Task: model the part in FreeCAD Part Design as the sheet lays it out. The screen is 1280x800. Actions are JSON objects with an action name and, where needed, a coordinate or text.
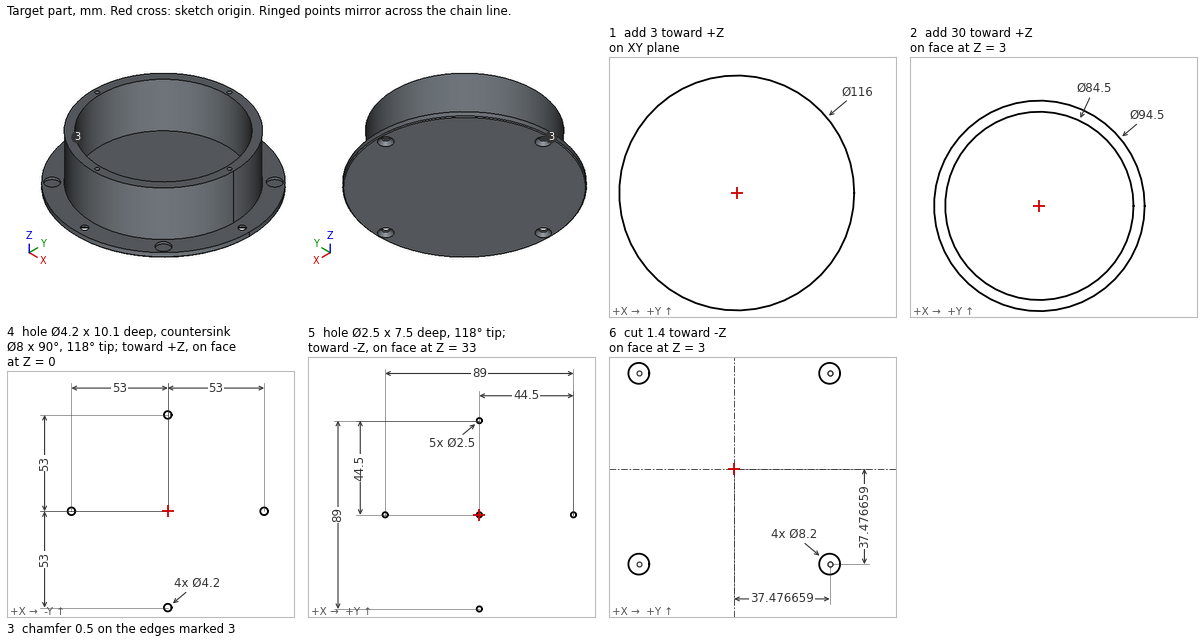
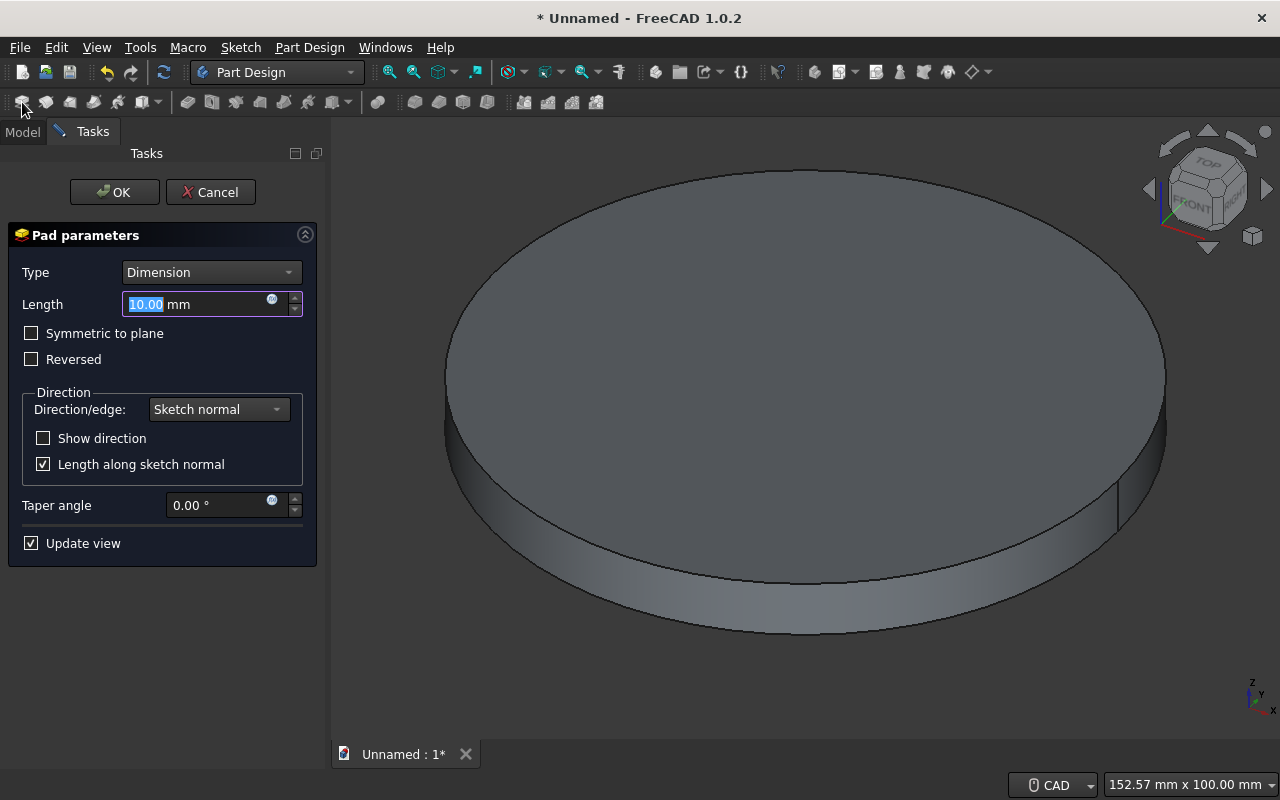
{"action": "type", "text": "3"}
{"action": "key", "text": "Tab"}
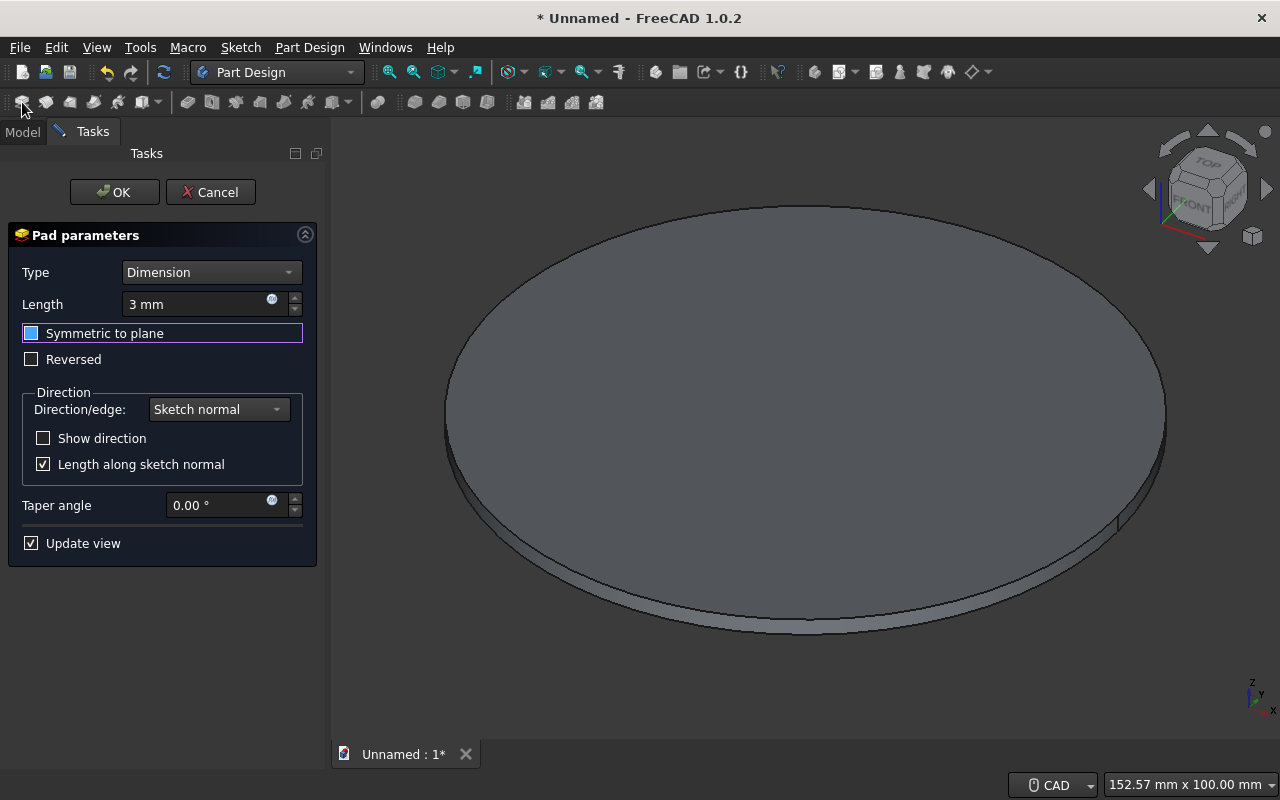
{"action": "left_click", "coordinate": [115, 192]}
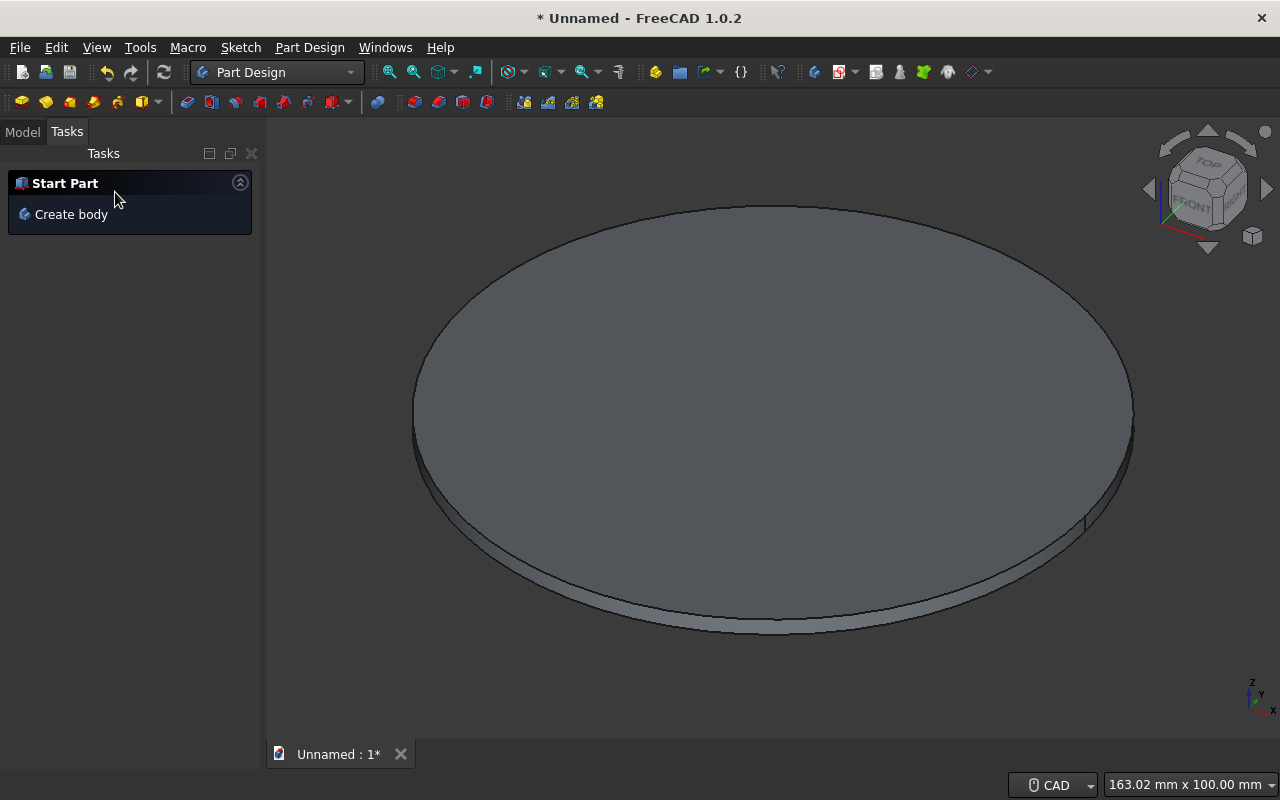
{"action": "left_click", "coordinate": [773, 412]}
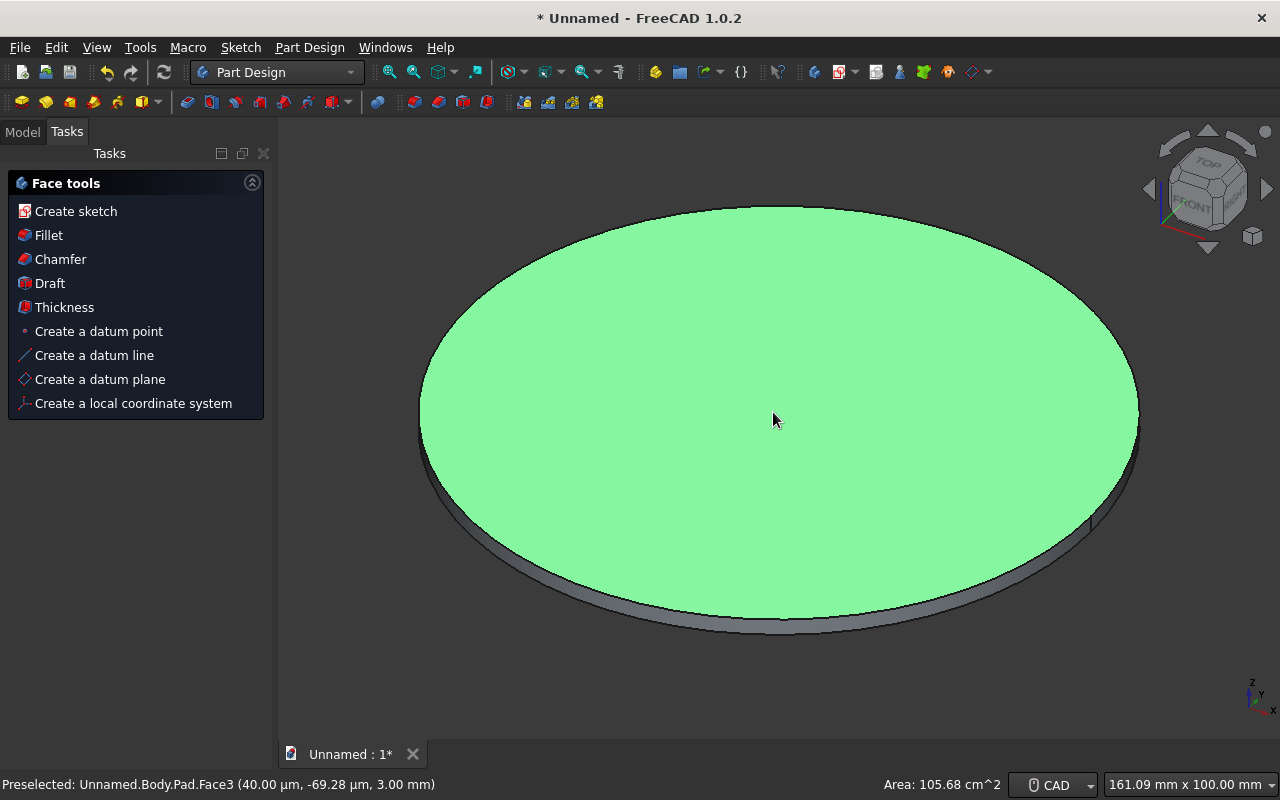
{"action": "left_click", "coordinate": [840, 72]}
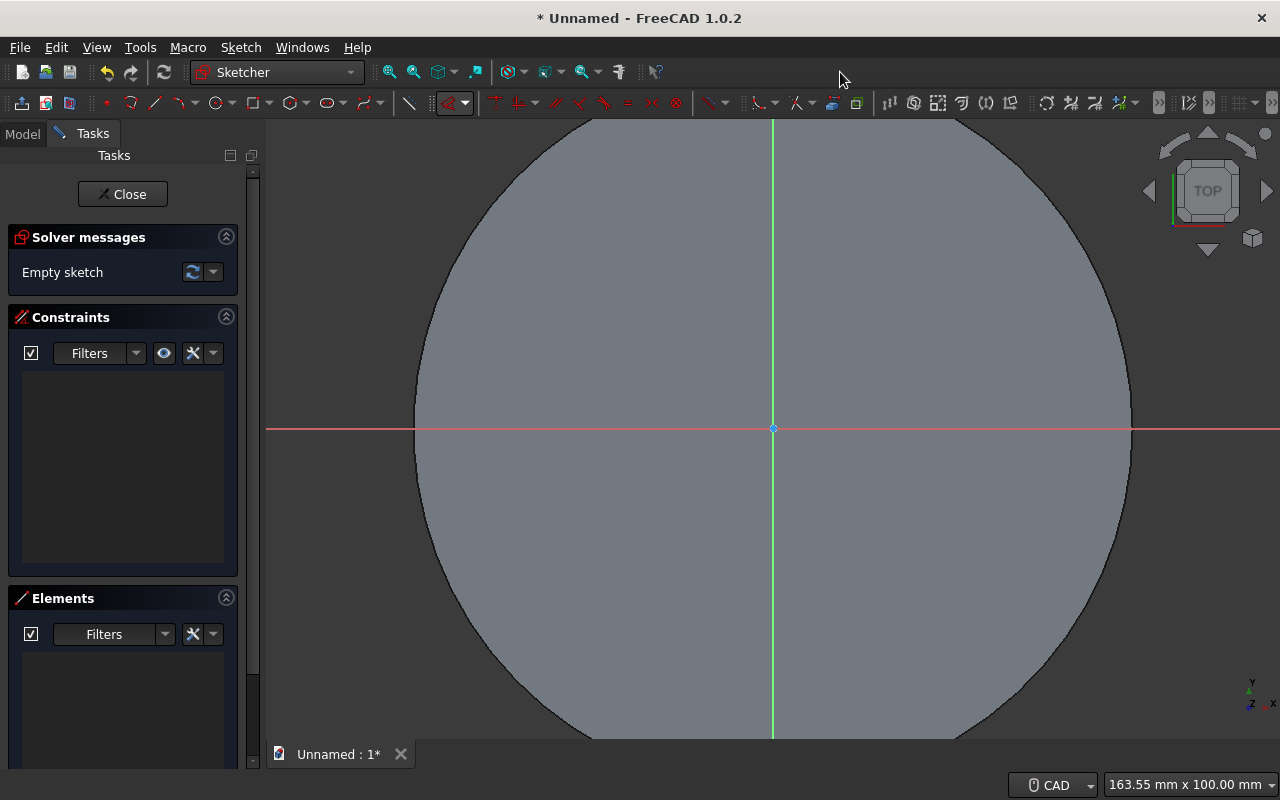
{"action": "scroll", "coordinate": [565, 429], "scroll_direction": "down", "scroll_amount": 2}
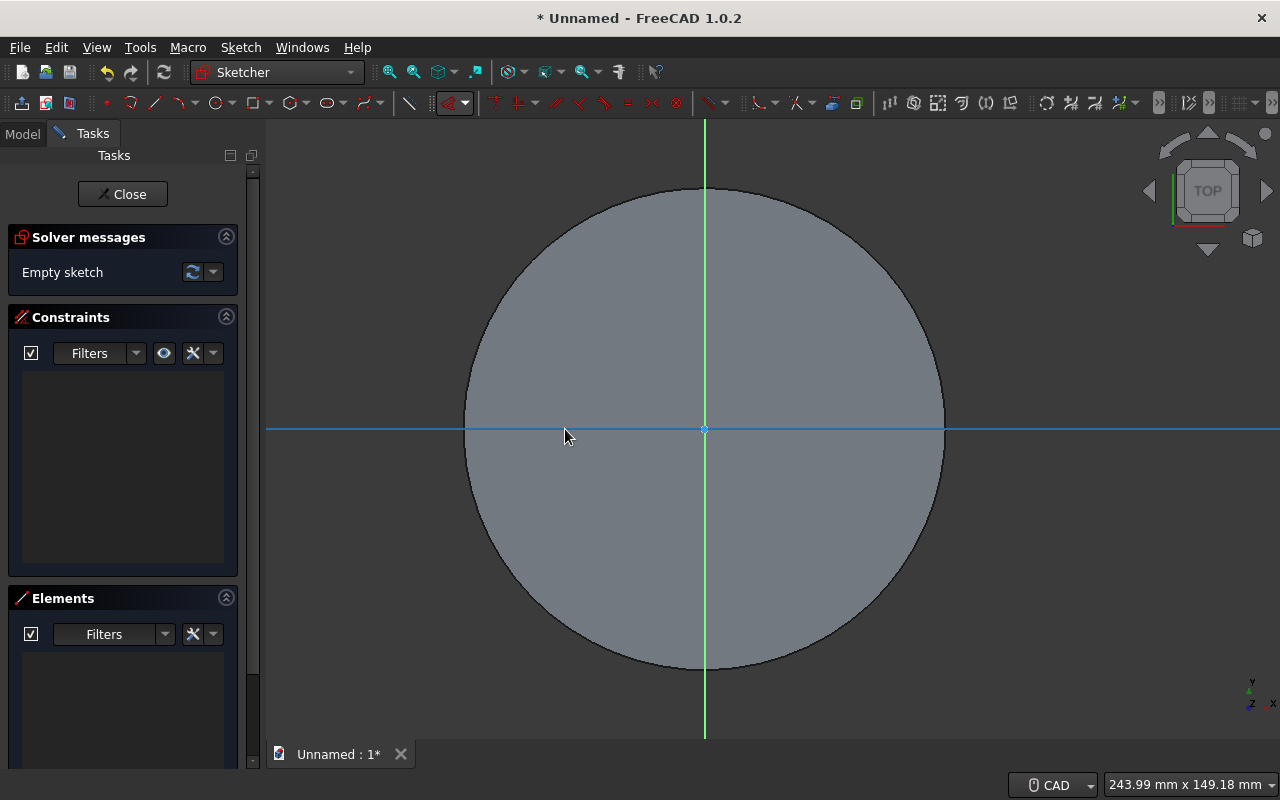
{"action": "left_click", "coordinate": [216, 104]}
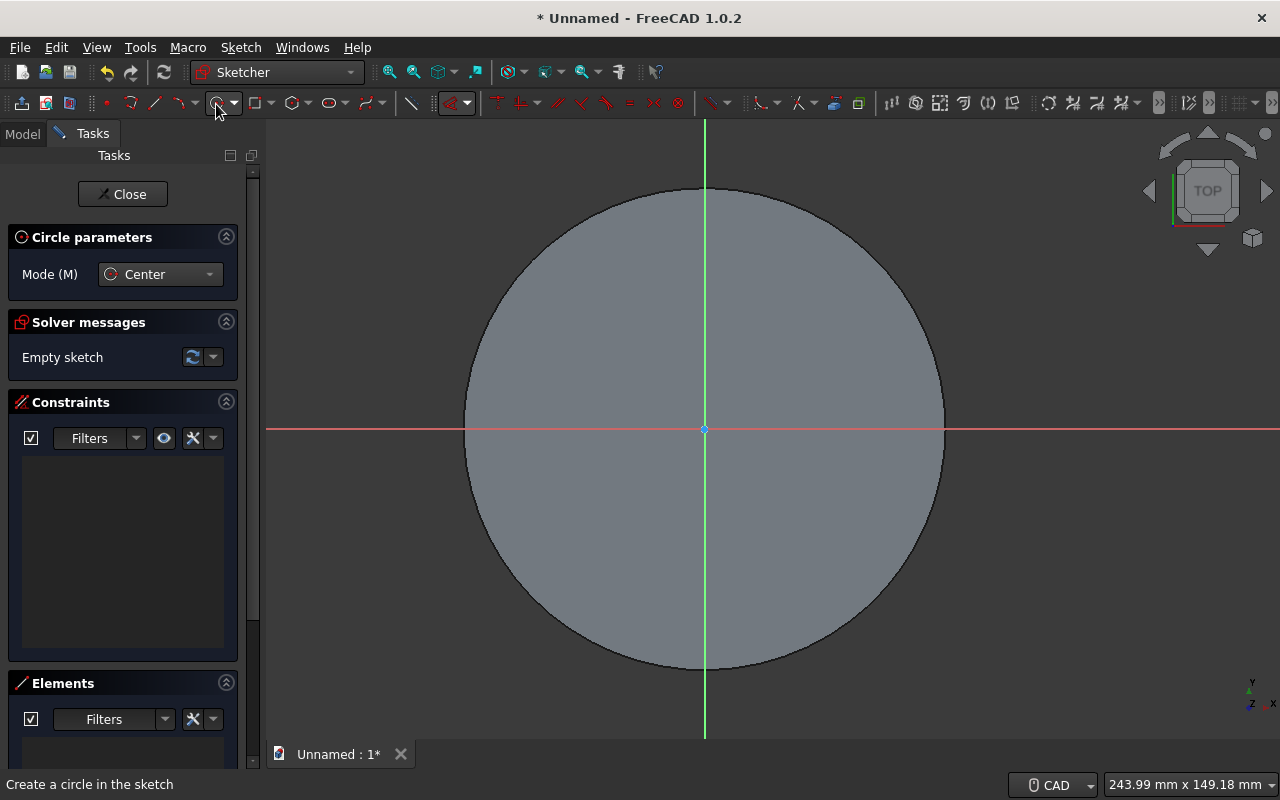
{"action": "left_click", "coordinate": [705, 429]}
{"action": "mouse_move", "coordinate": [843, 290]}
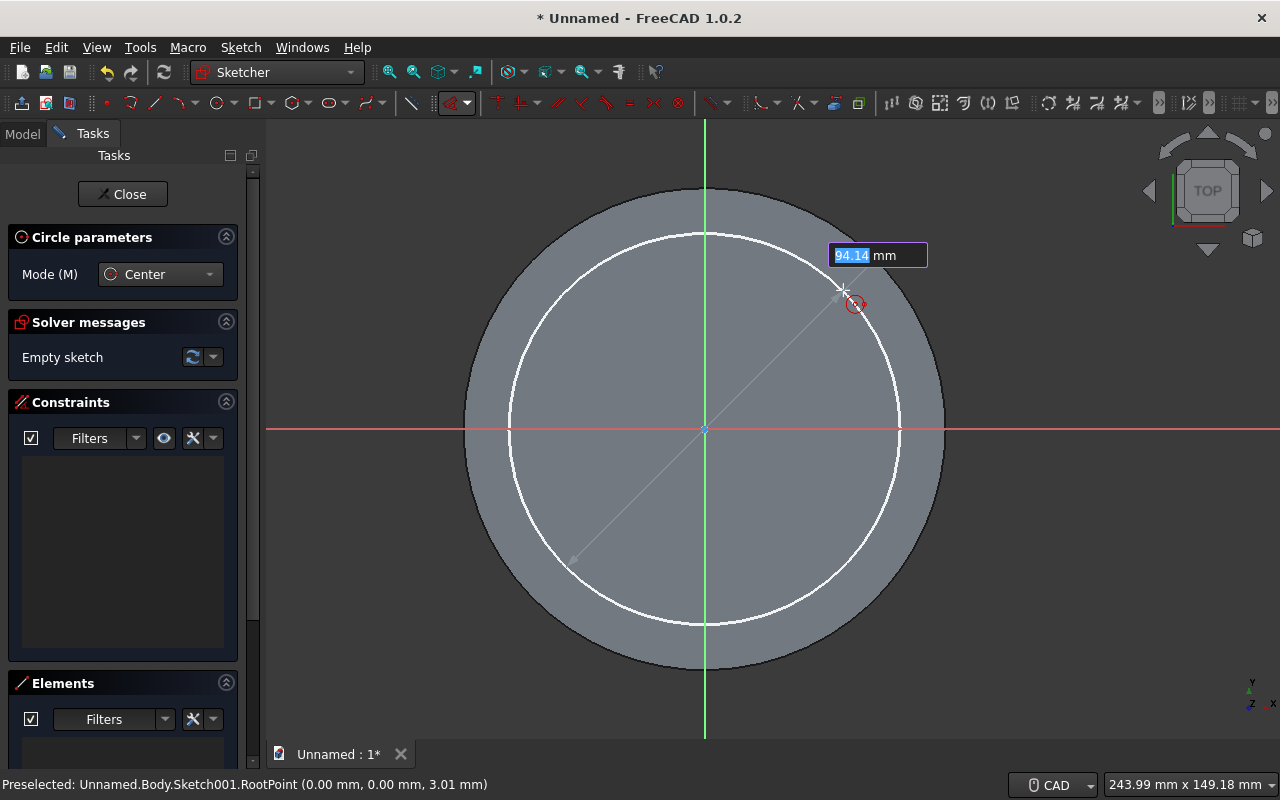
{"action": "type", "text": "94.5"}
{"action": "key", "text": "Return"}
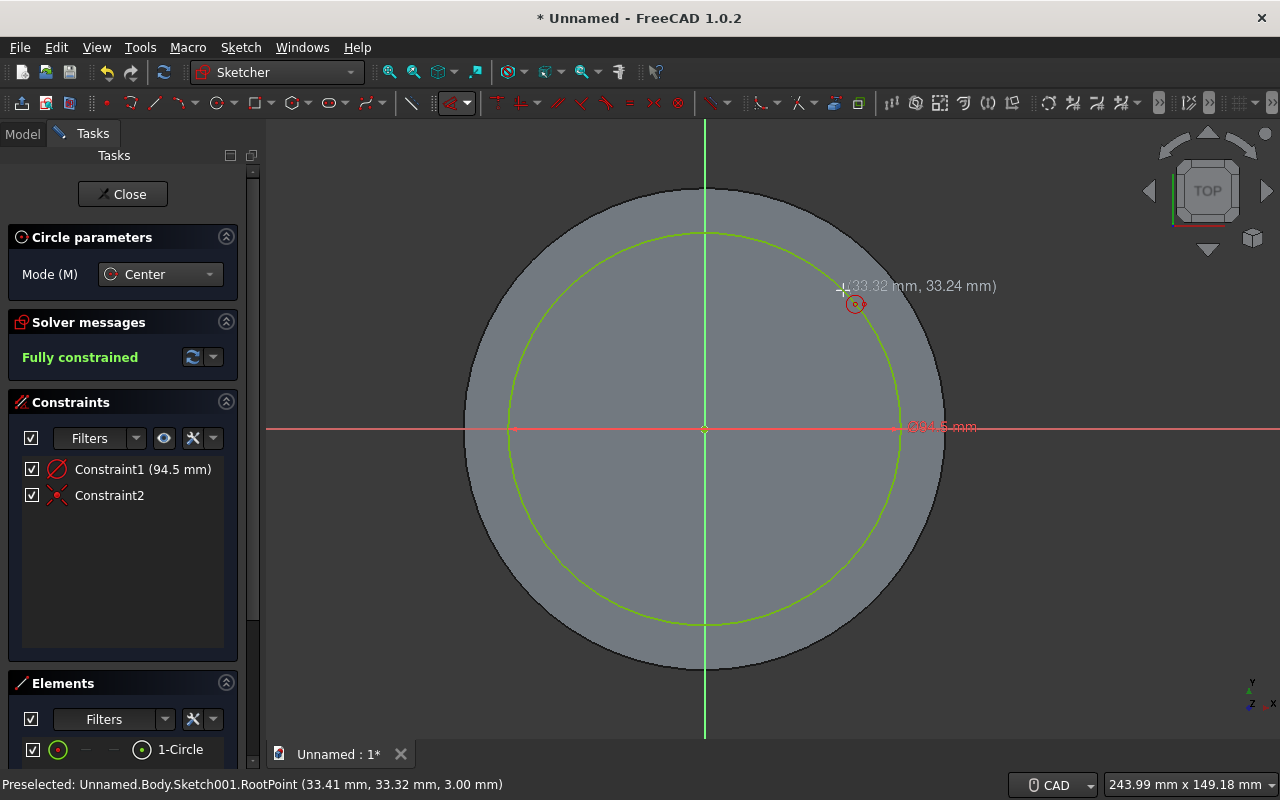
{"action": "left_click", "coordinate": [705, 429]}
{"action": "mouse_move", "coordinate": [829, 305]}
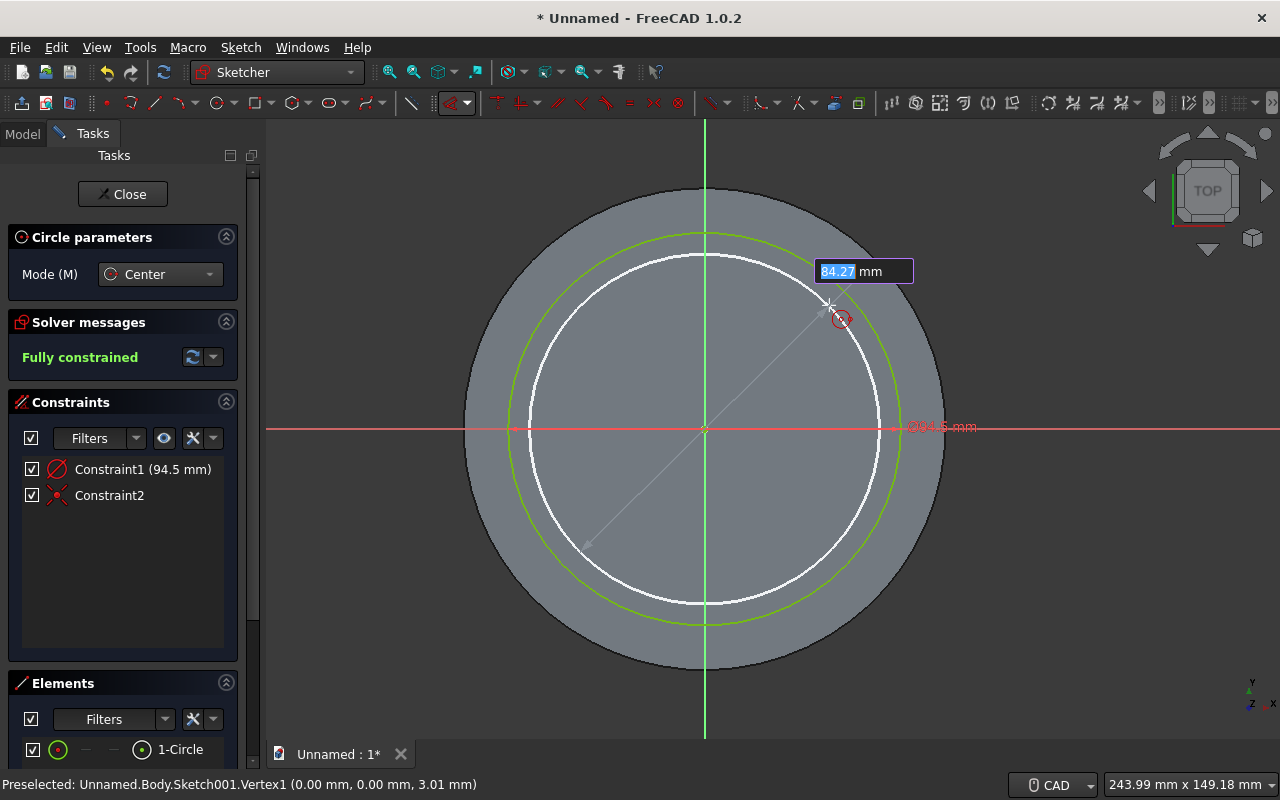
{"action": "type", "text": "84.5"}
{"action": "key", "text": "Return"}
{"action": "key", "text": "Escape"}